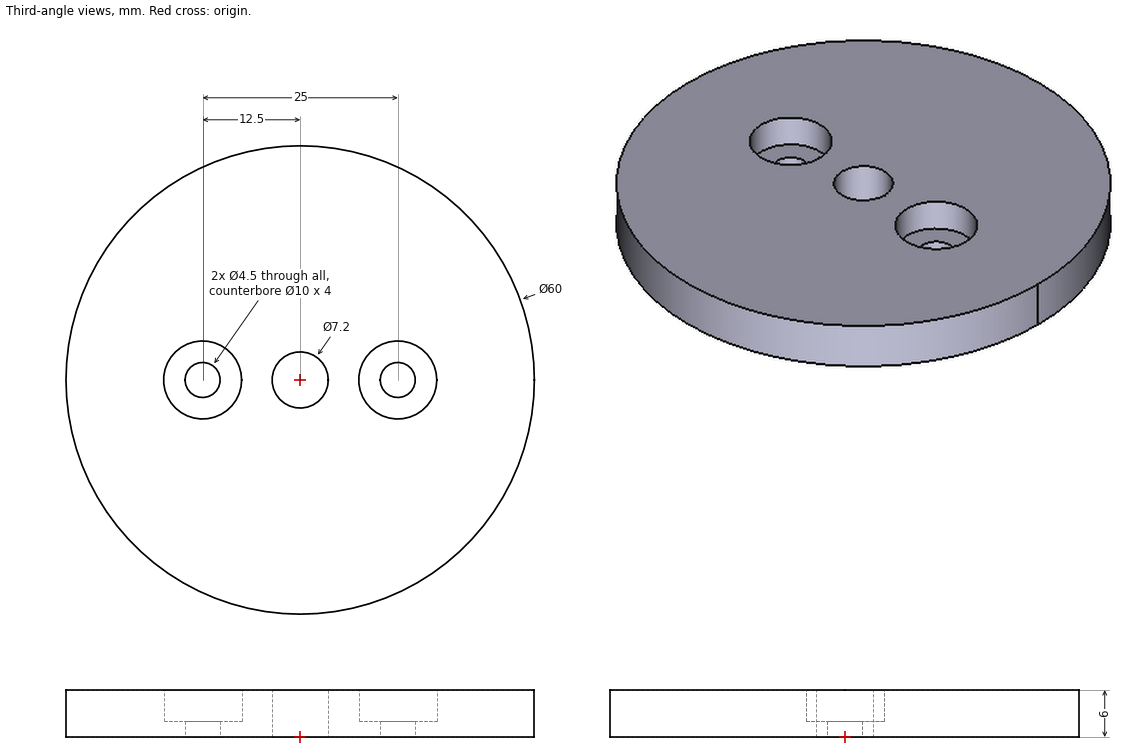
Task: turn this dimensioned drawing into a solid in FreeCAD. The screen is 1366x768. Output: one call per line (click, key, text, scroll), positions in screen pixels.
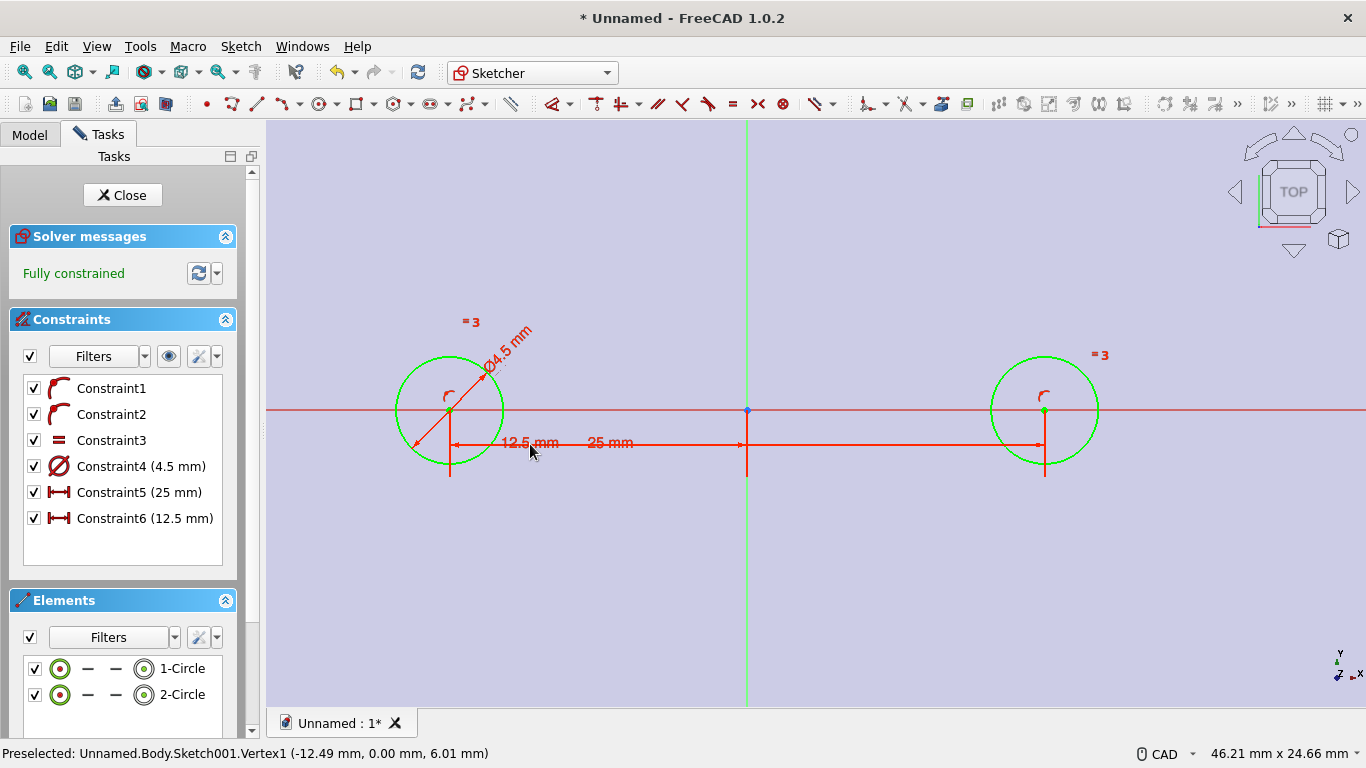
click(123, 195)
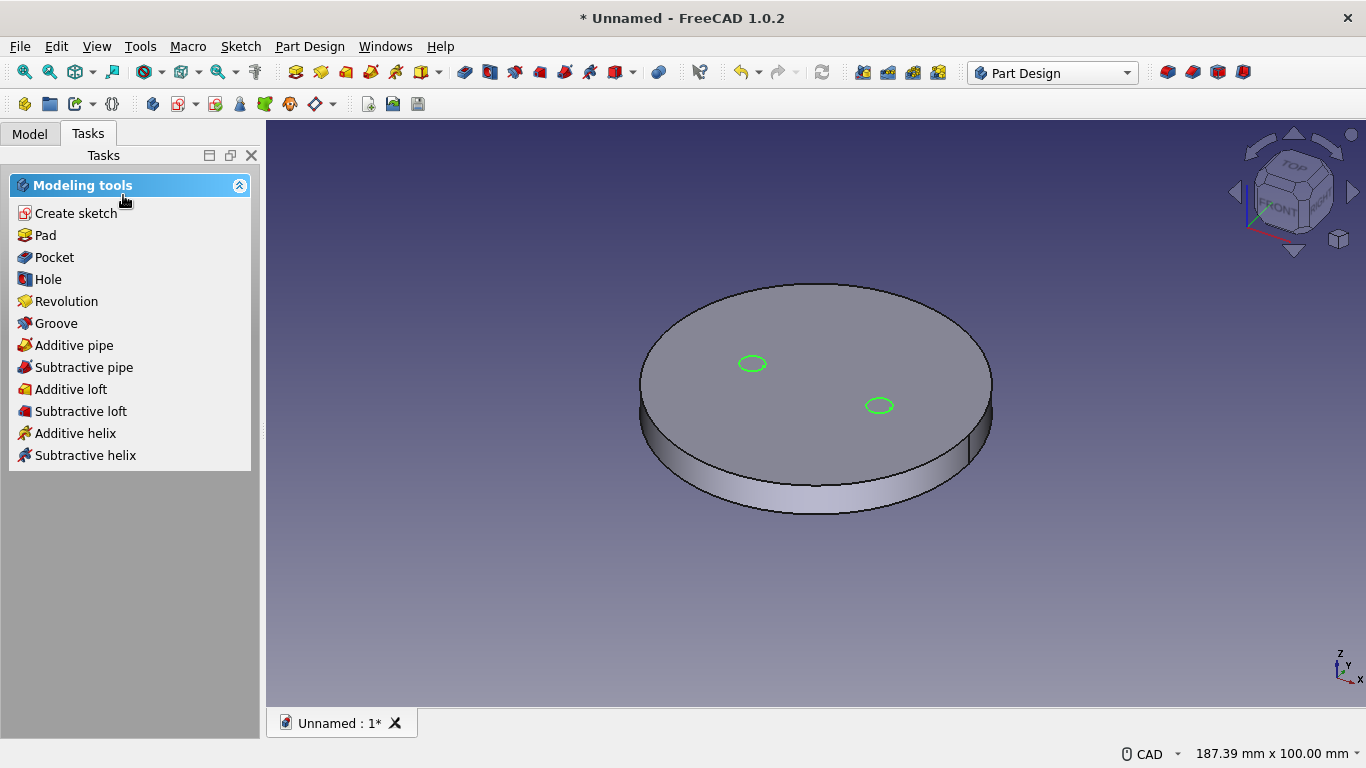
click(490, 72)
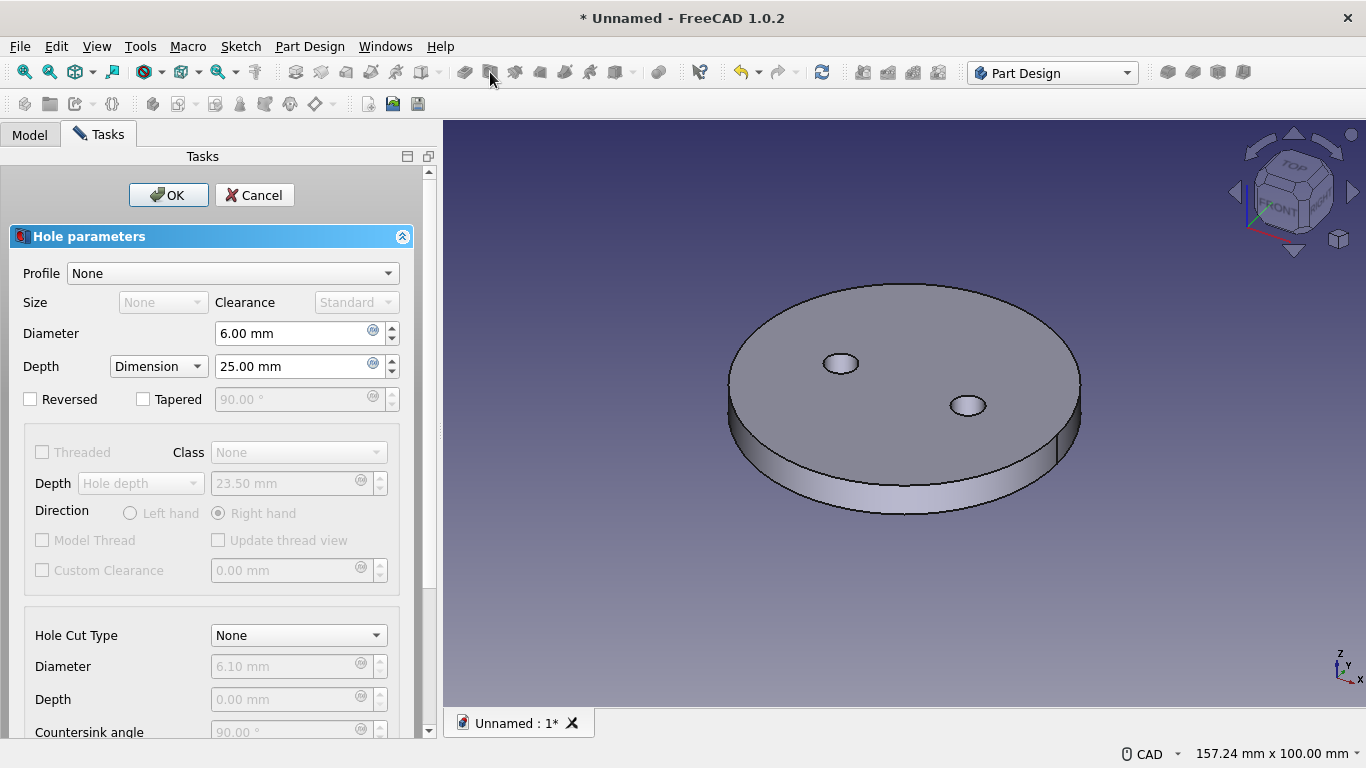
triple_click(300, 334)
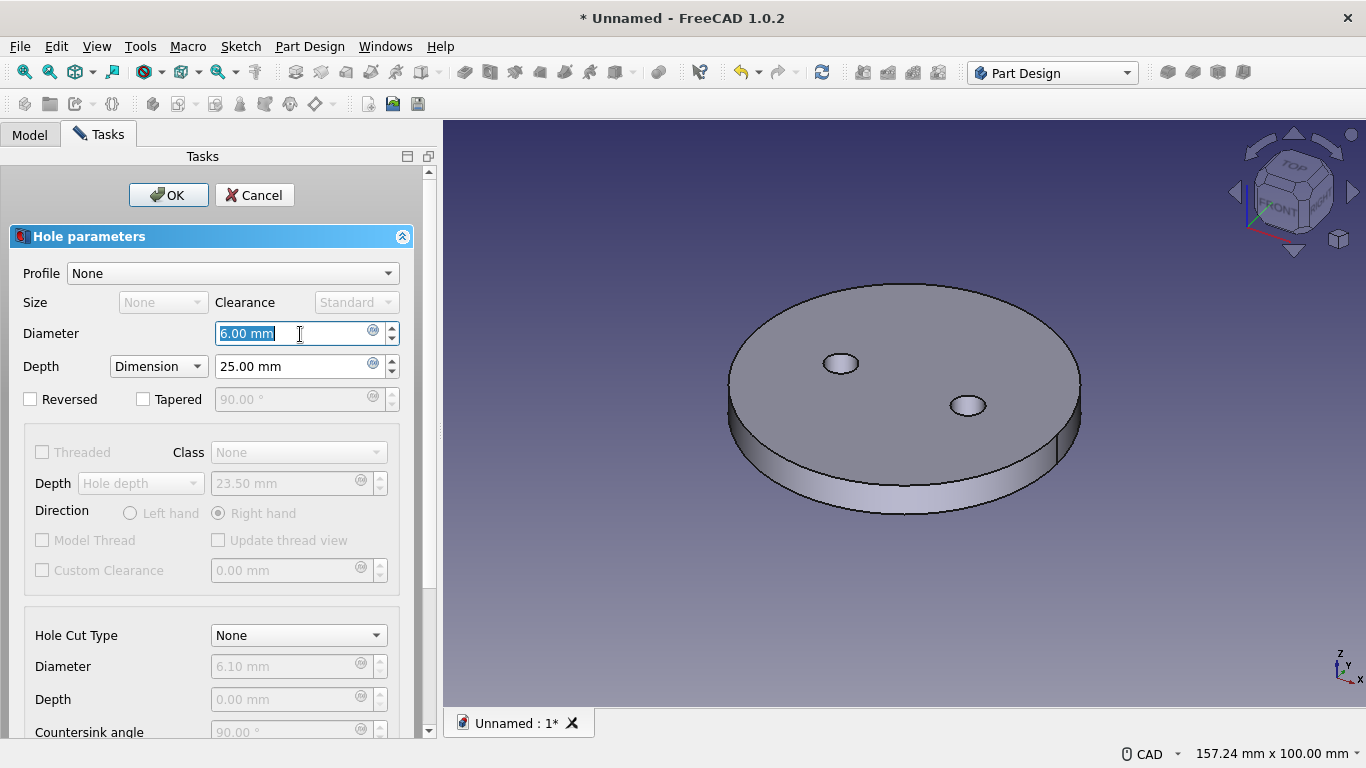
text(4.5)
key(Tab)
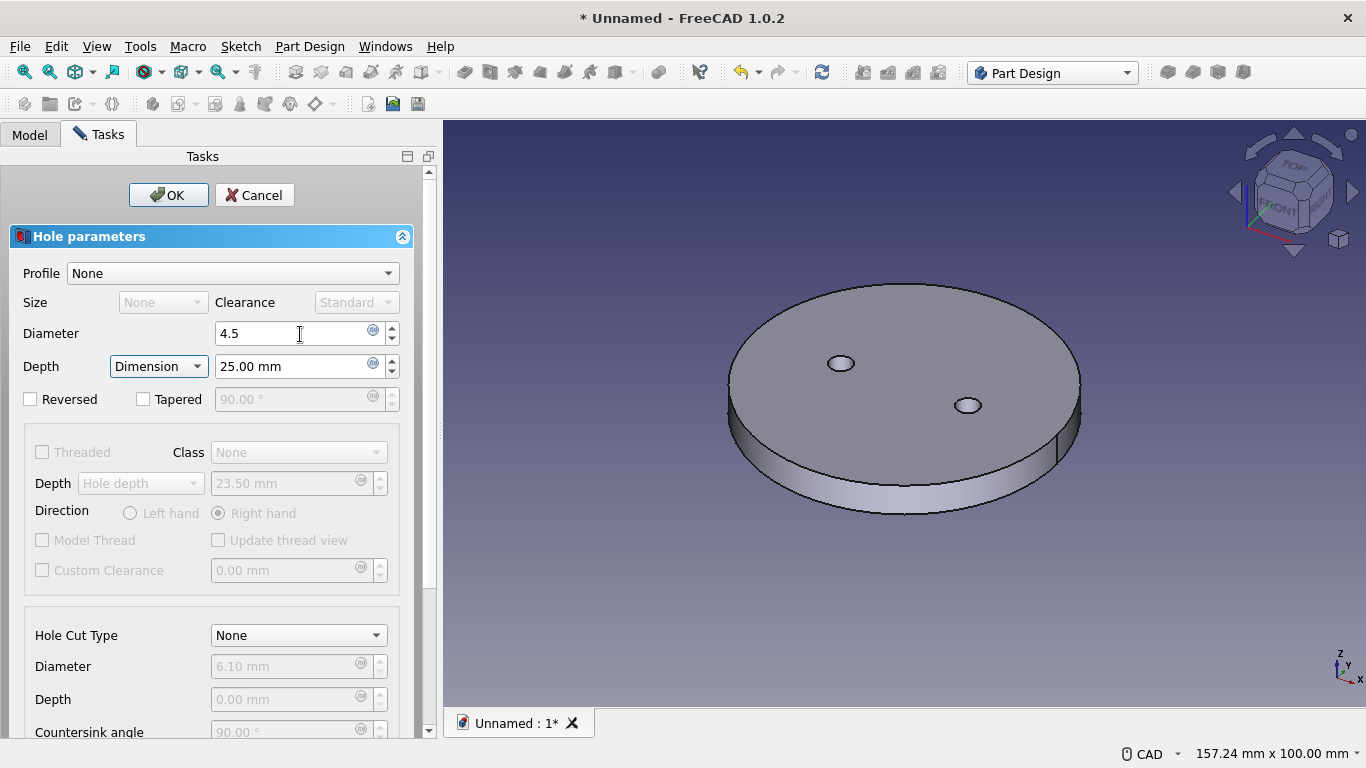
click(160, 366)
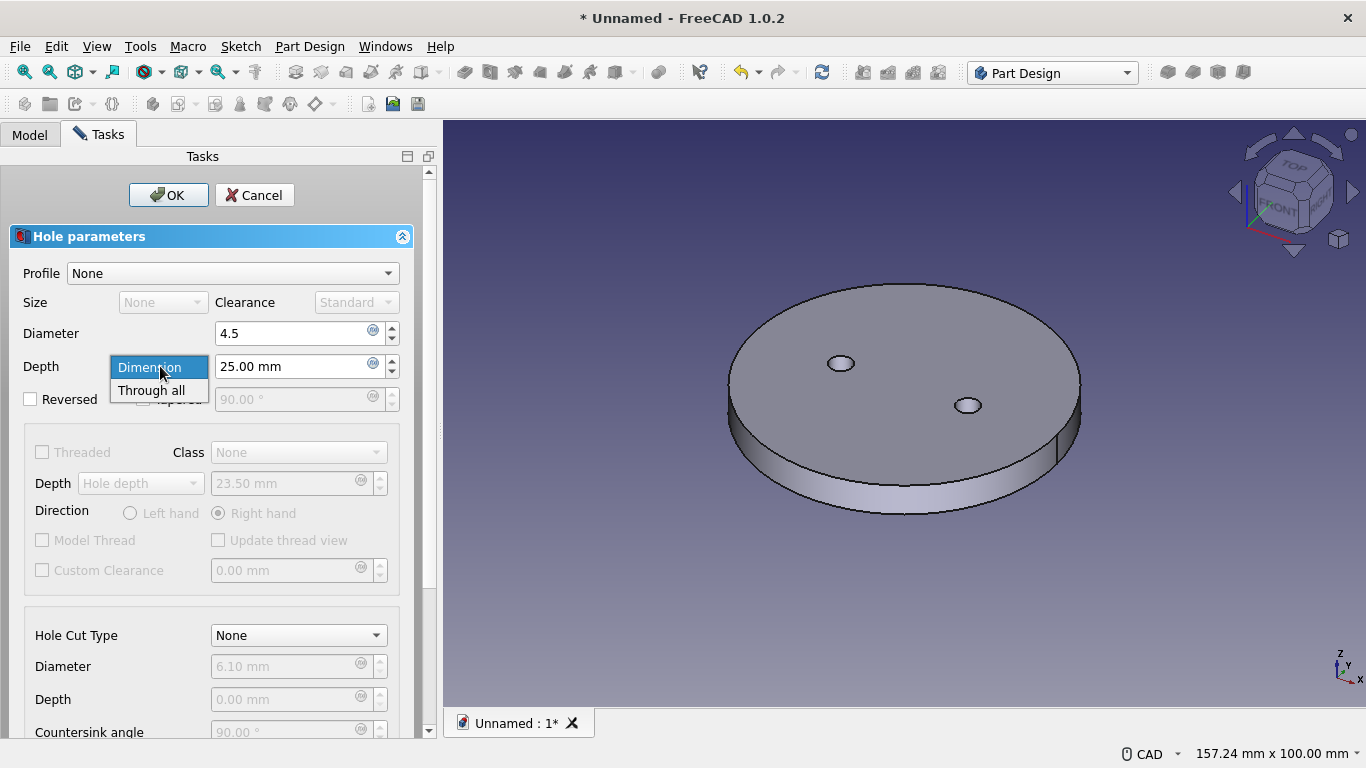
click(158, 390)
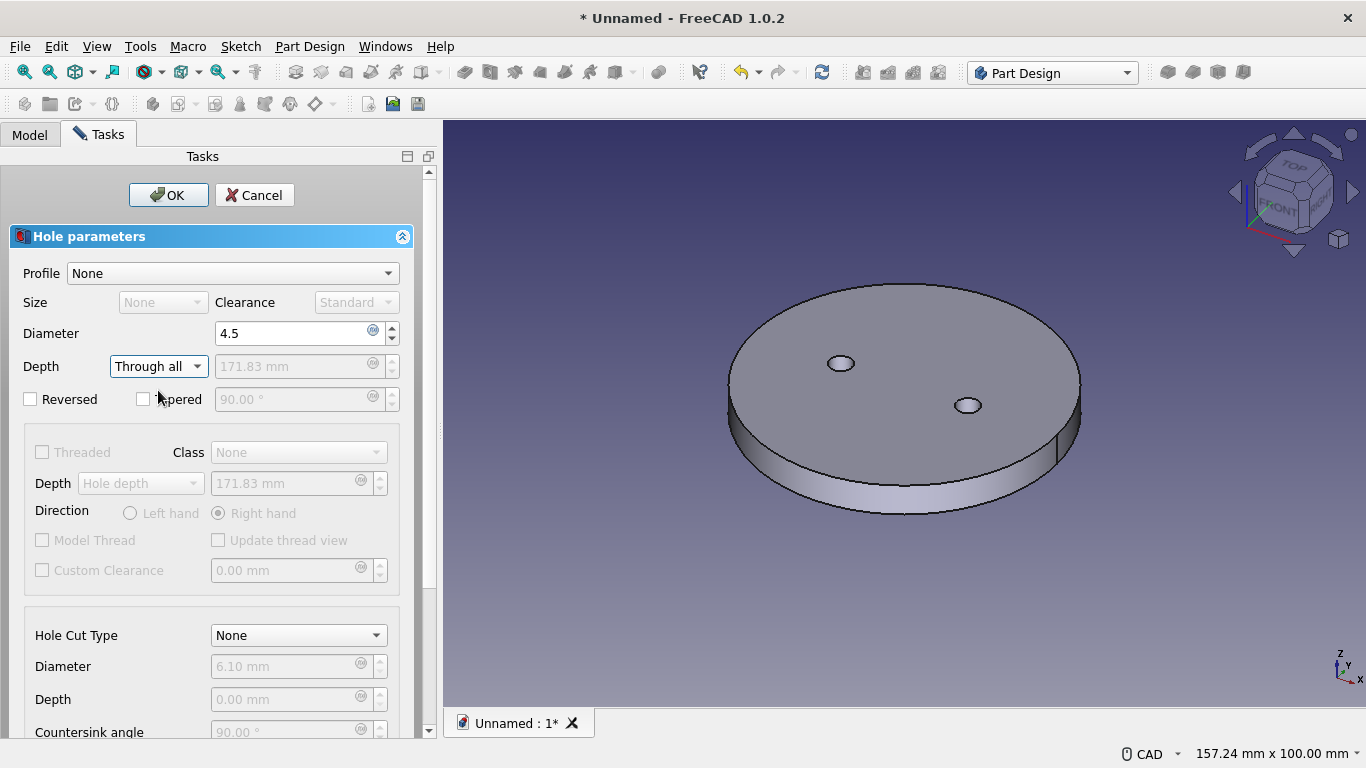
click(300, 636)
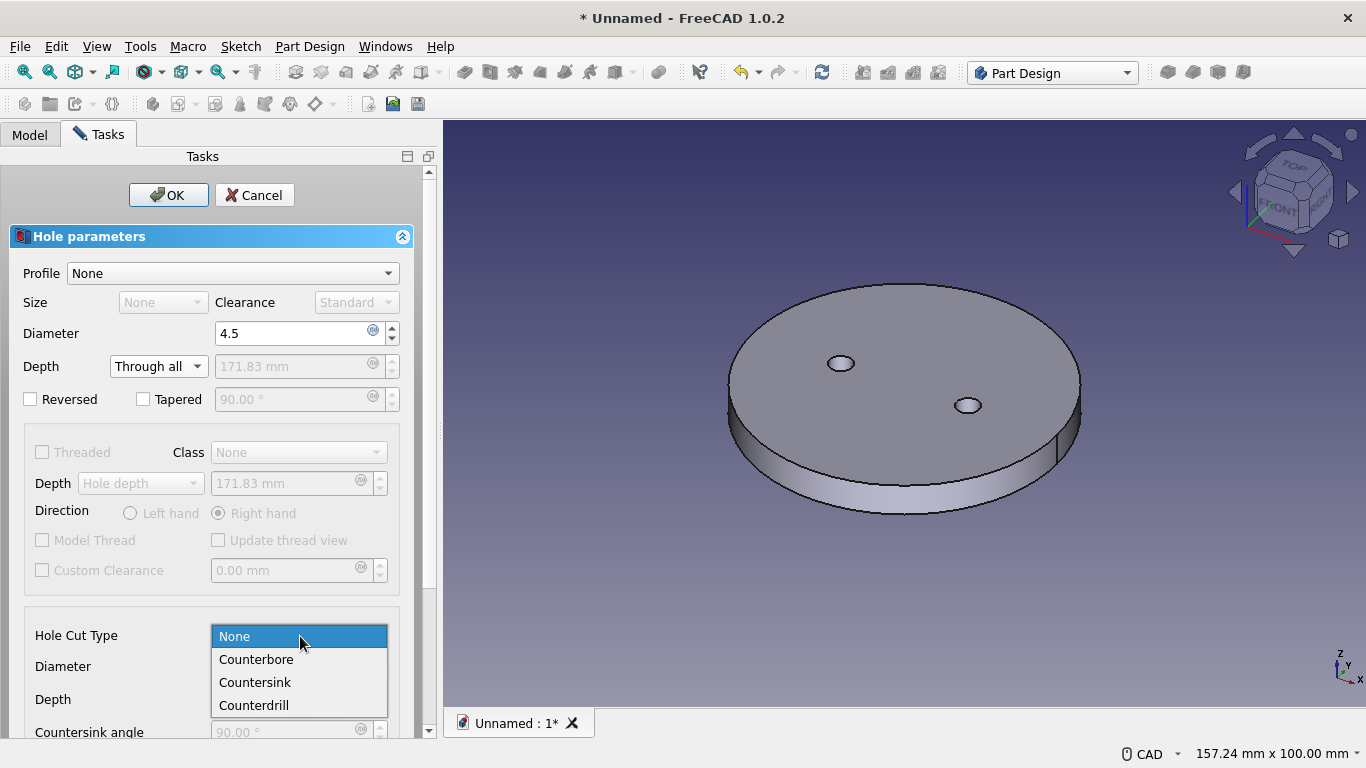
click(298, 660)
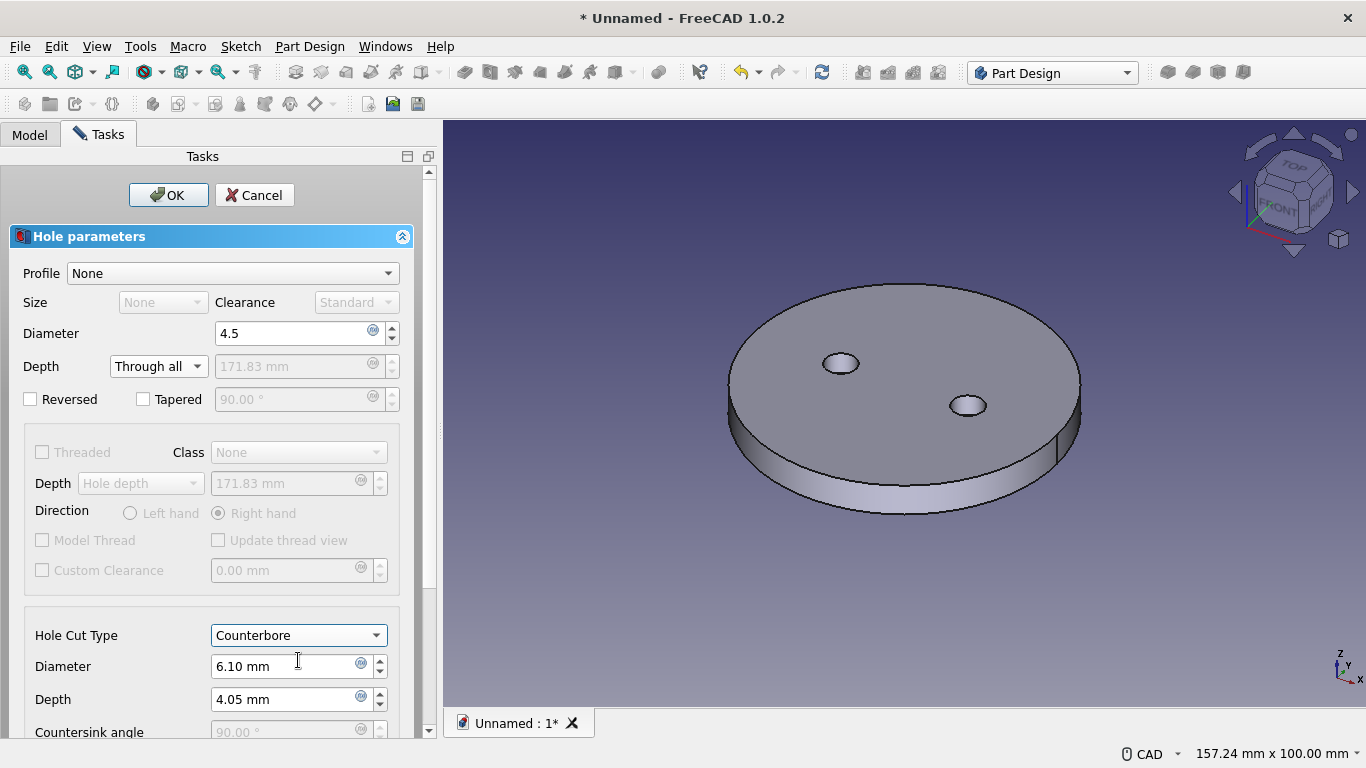
triple_click(292, 666)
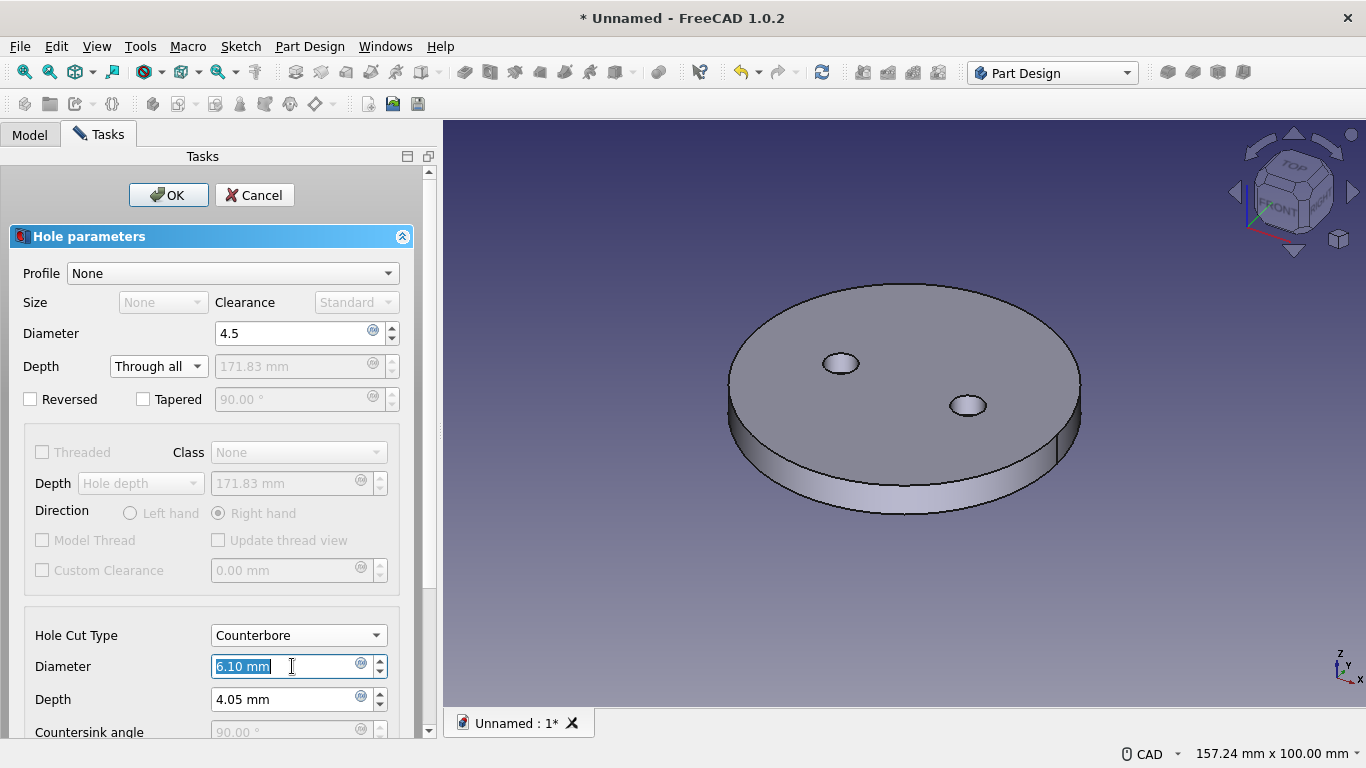
text(10)
key(Tab)